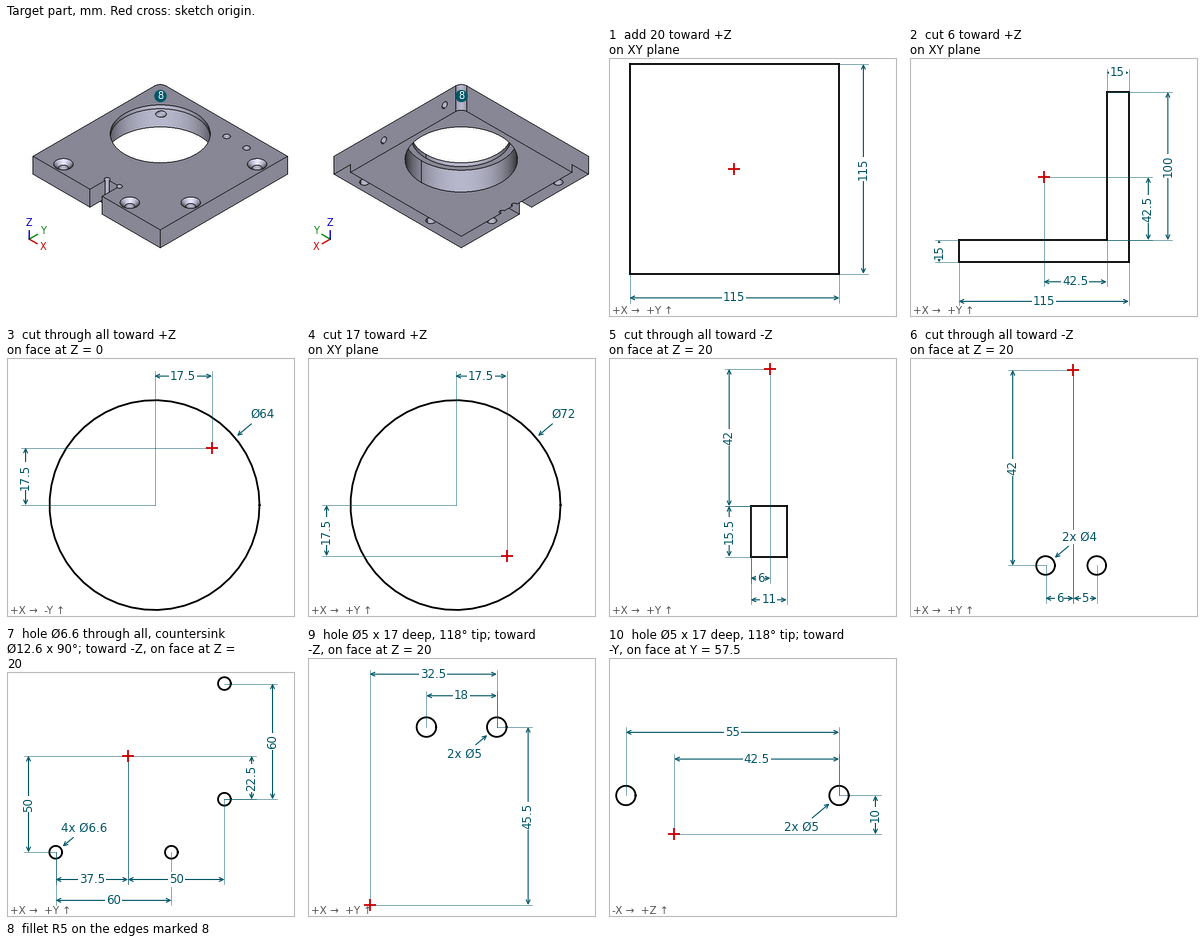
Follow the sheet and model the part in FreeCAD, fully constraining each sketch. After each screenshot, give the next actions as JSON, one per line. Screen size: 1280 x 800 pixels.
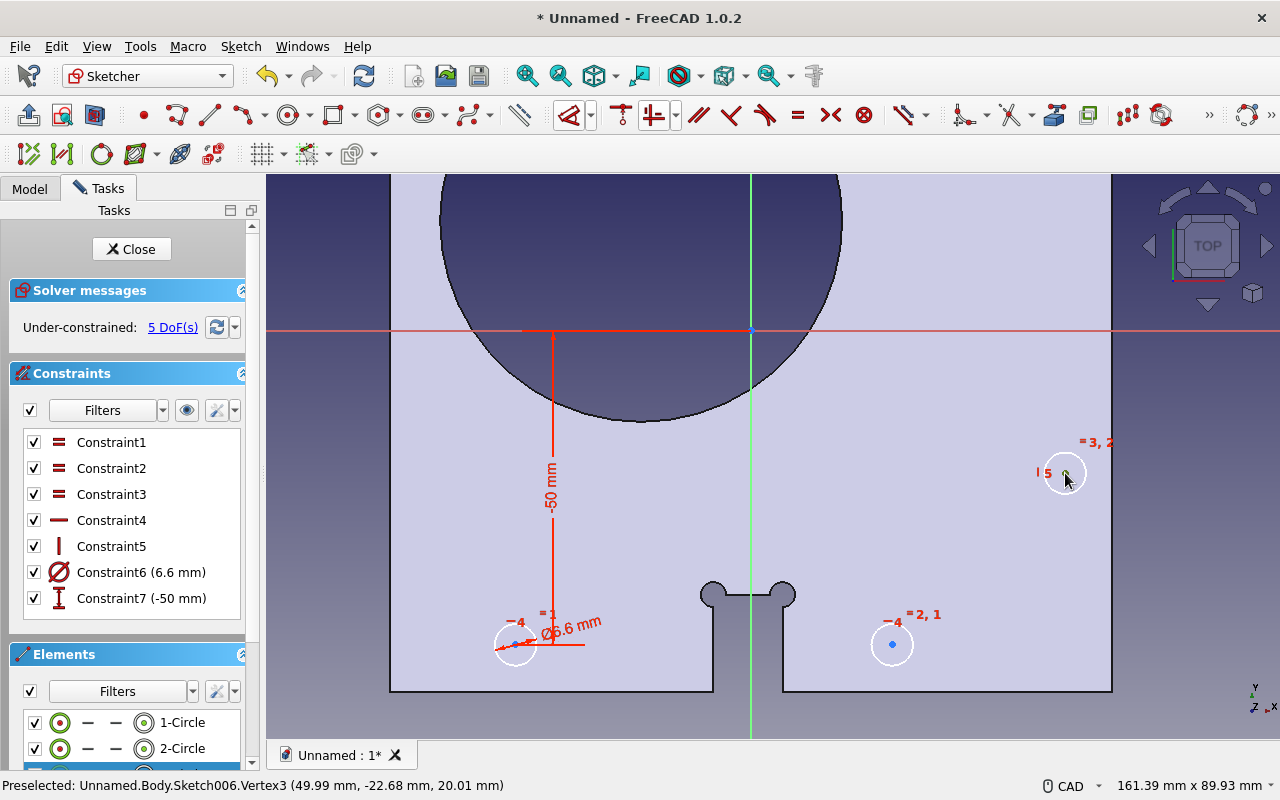
{"action": "key", "text": "l"}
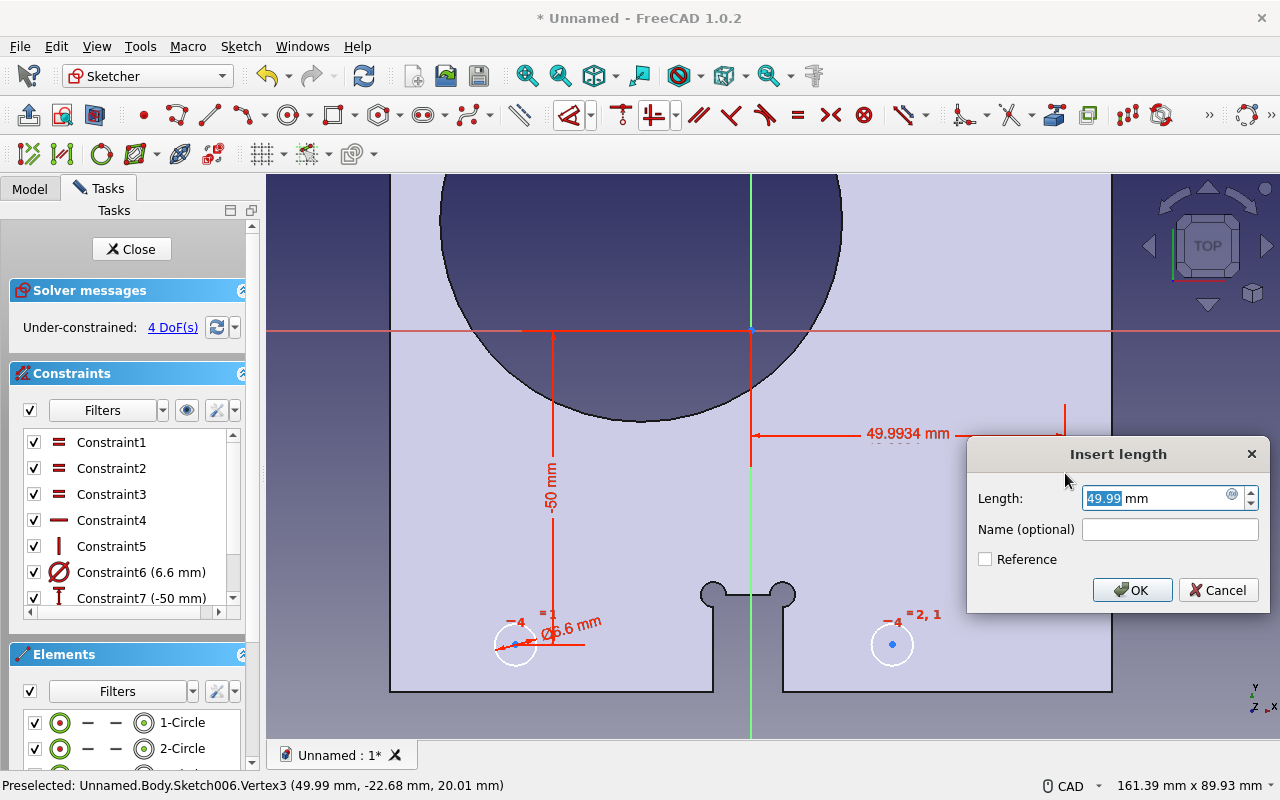
{"action": "type", "text": "50"}
{"action": "key", "text": "Return"}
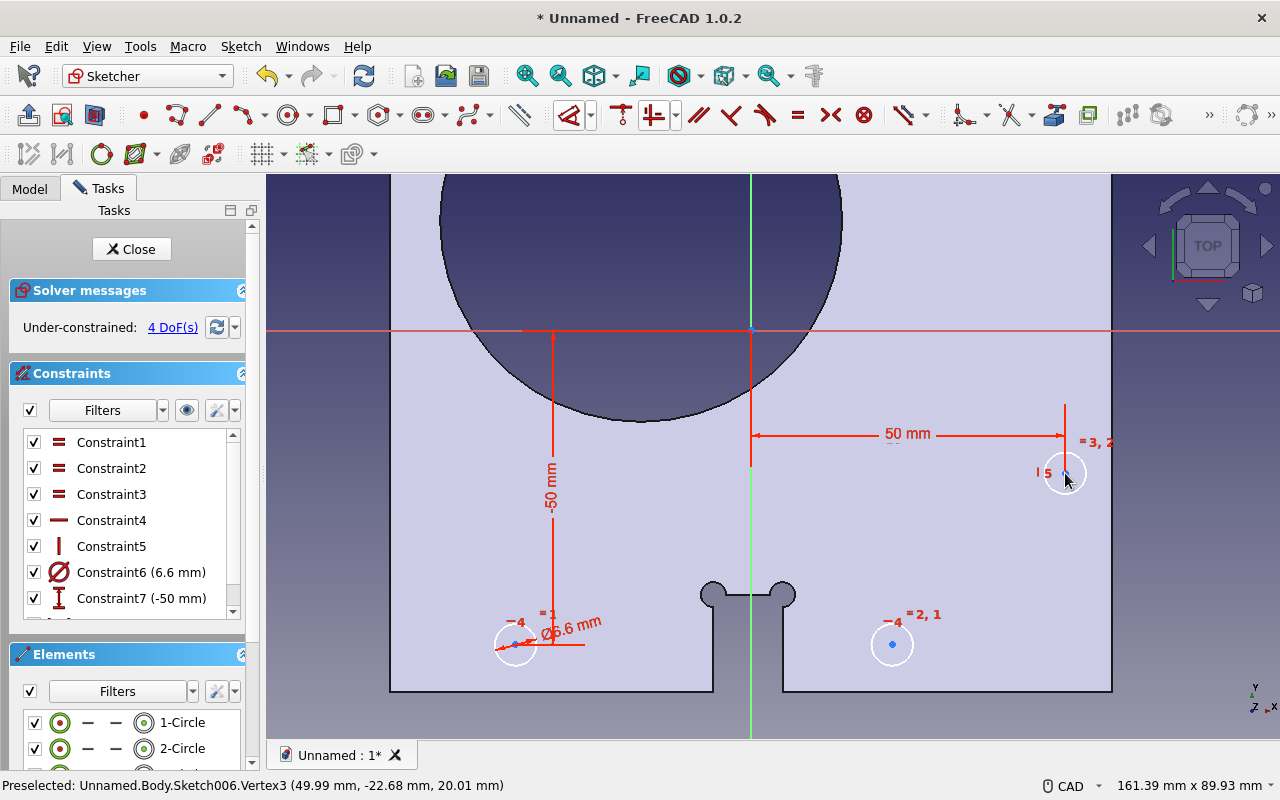
{"action": "left_click", "coordinate": [516, 645]}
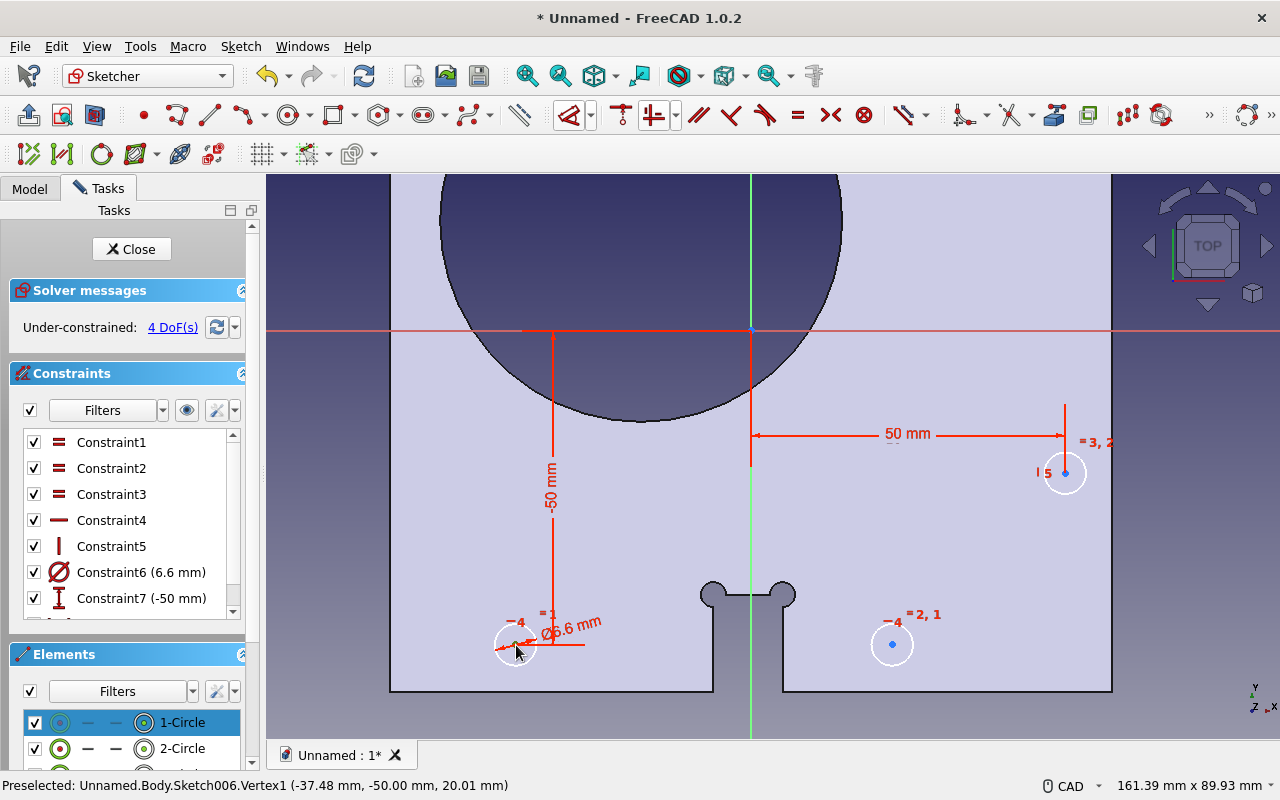
{"action": "left_click", "coordinate": [892, 645]}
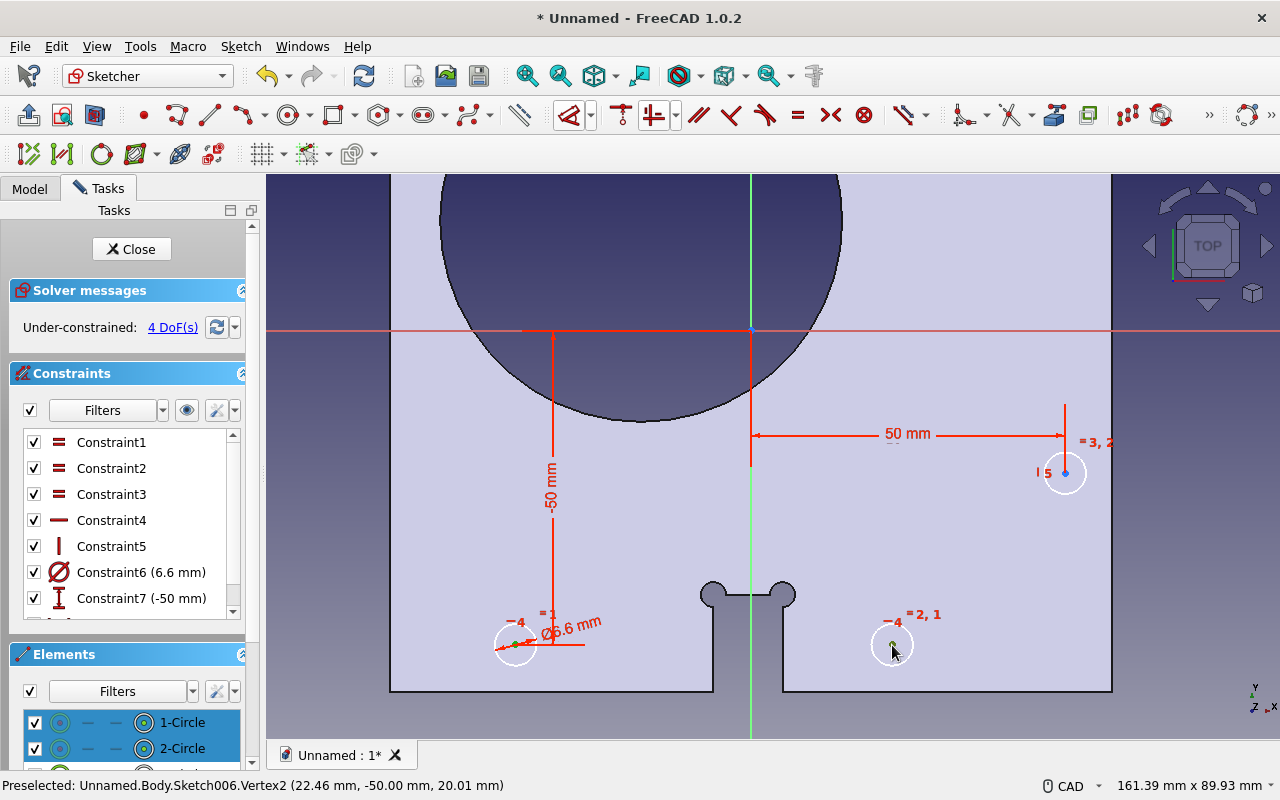
{"action": "left_click", "coordinate": [590, 116]}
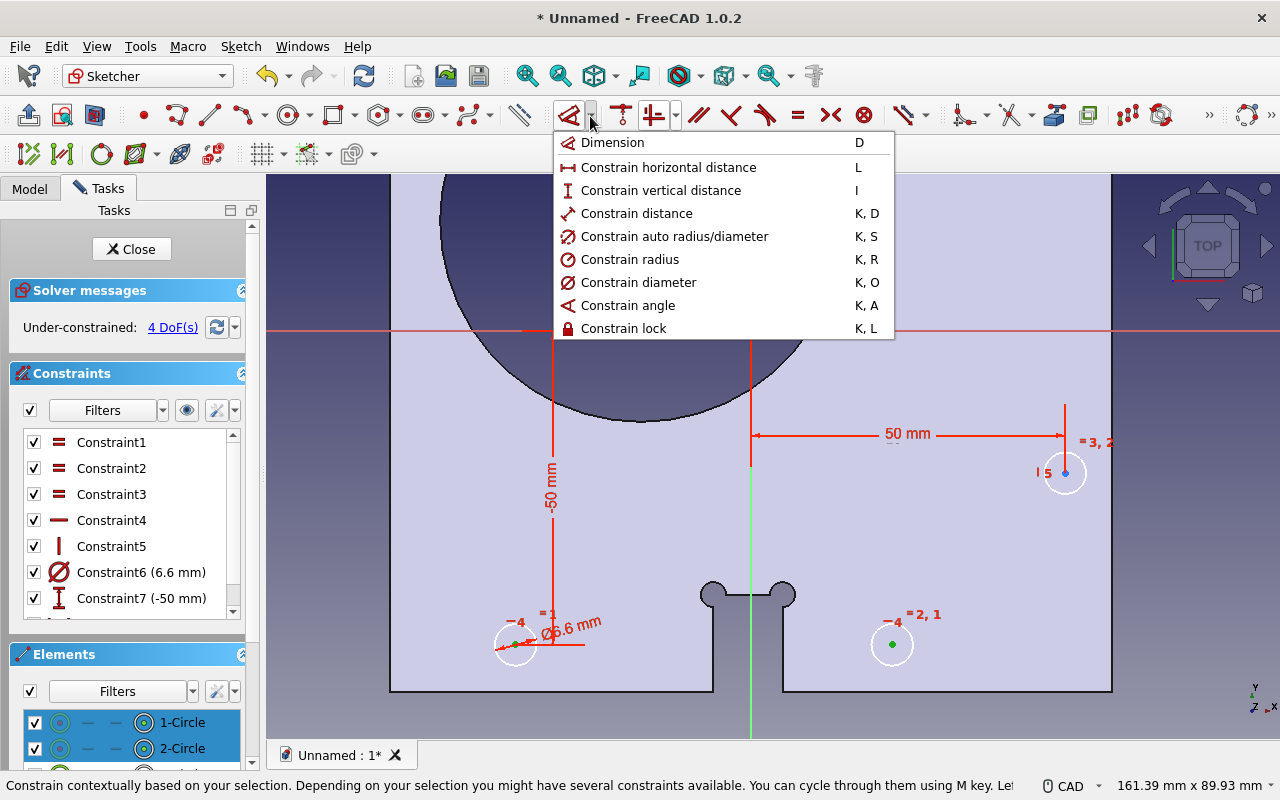
{"action": "left_click", "coordinate": [724, 168]}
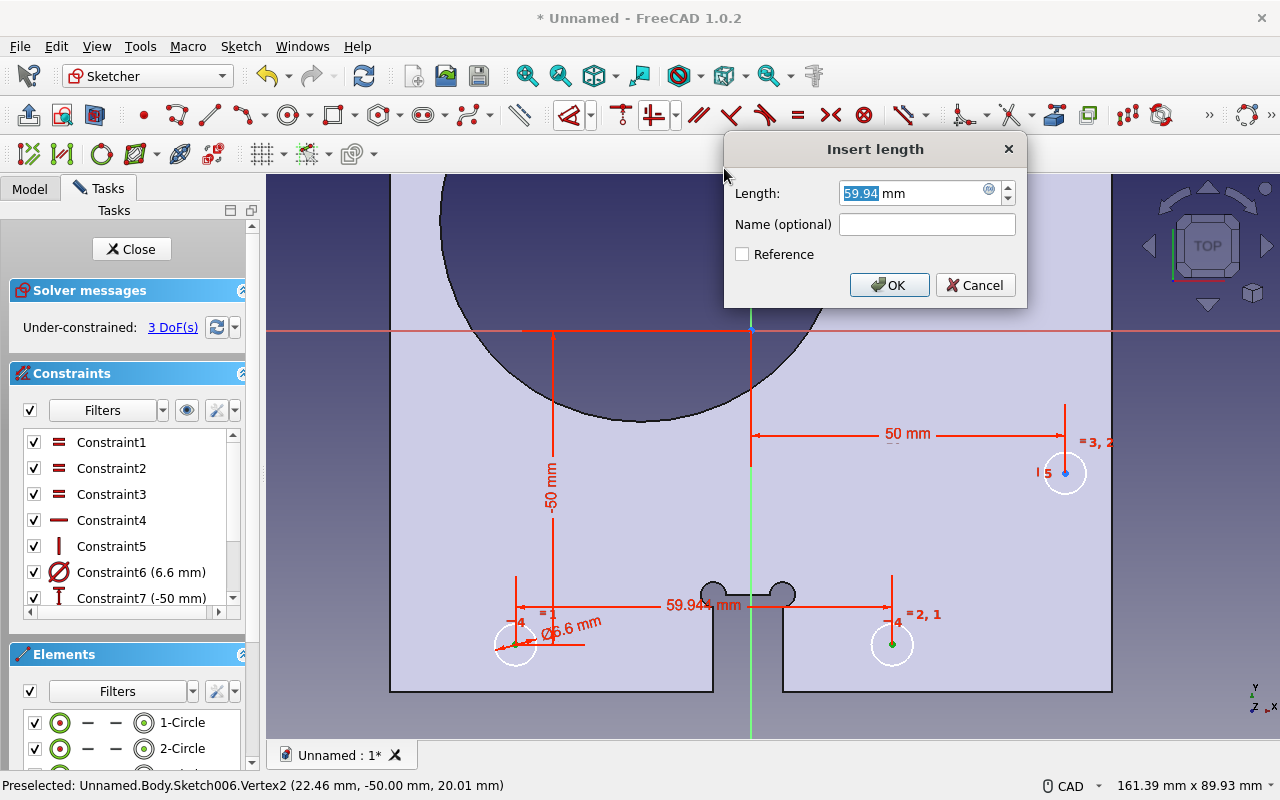
{"action": "type", "text": "60"}
{"action": "key", "text": "Return"}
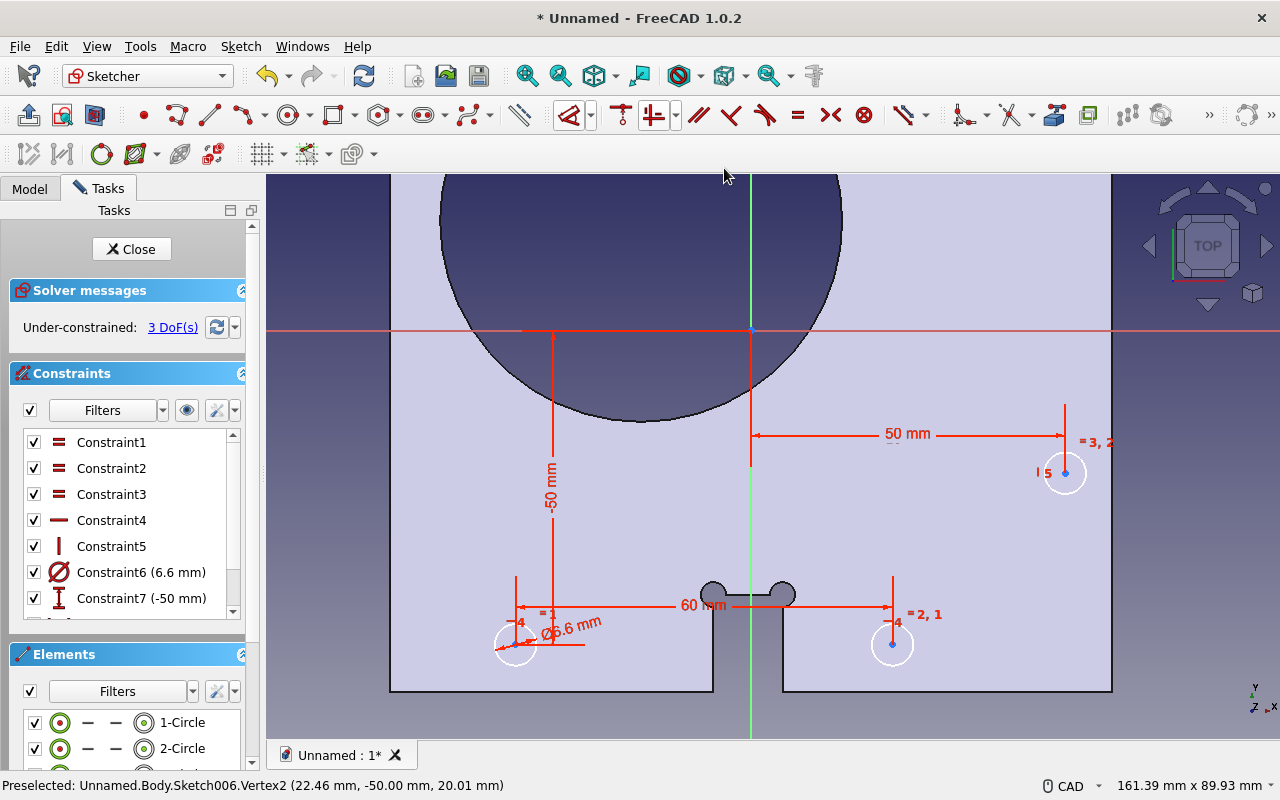
{"action": "left_click", "coordinate": [1065, 473]}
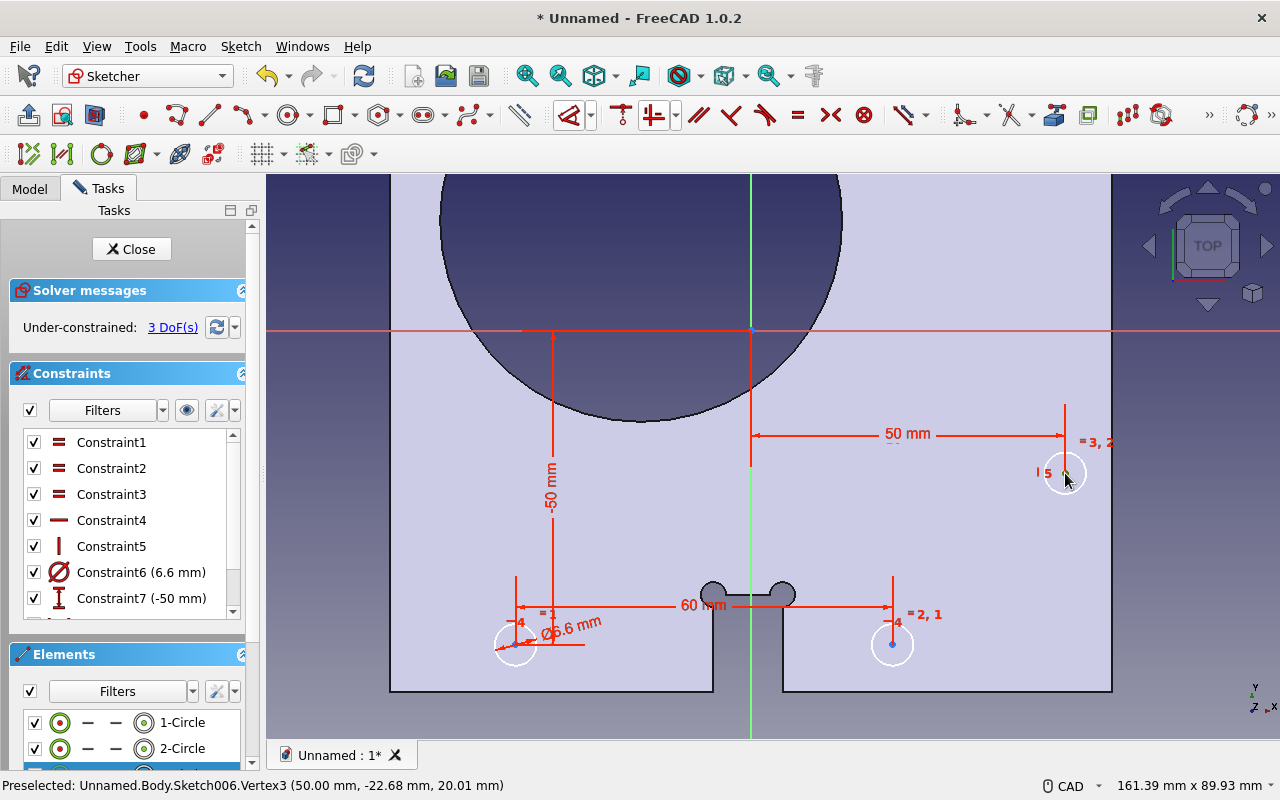
{"action": "scroll", "coordinate": [530, 632], "scroll_direction": "down", "scroll_amount": 2}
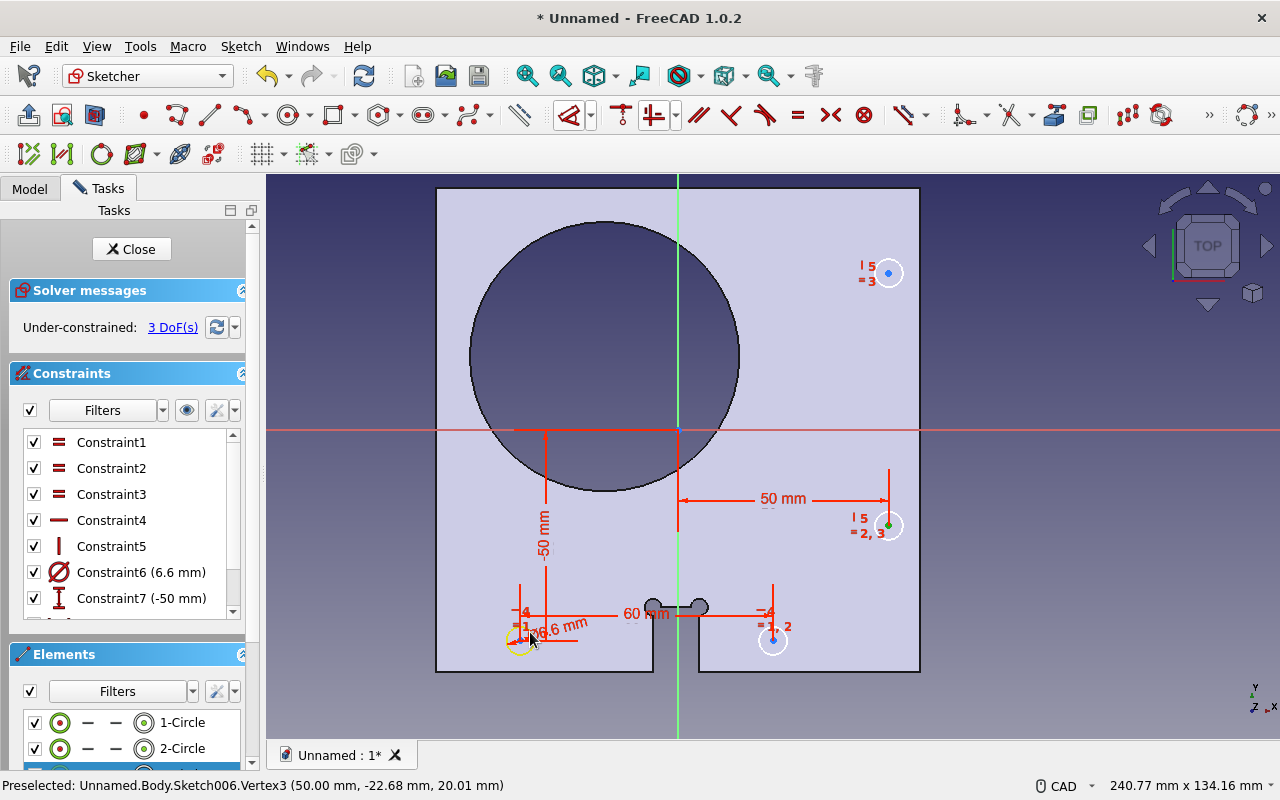
{"action": "left_click", "coordinate": [889, 273]}